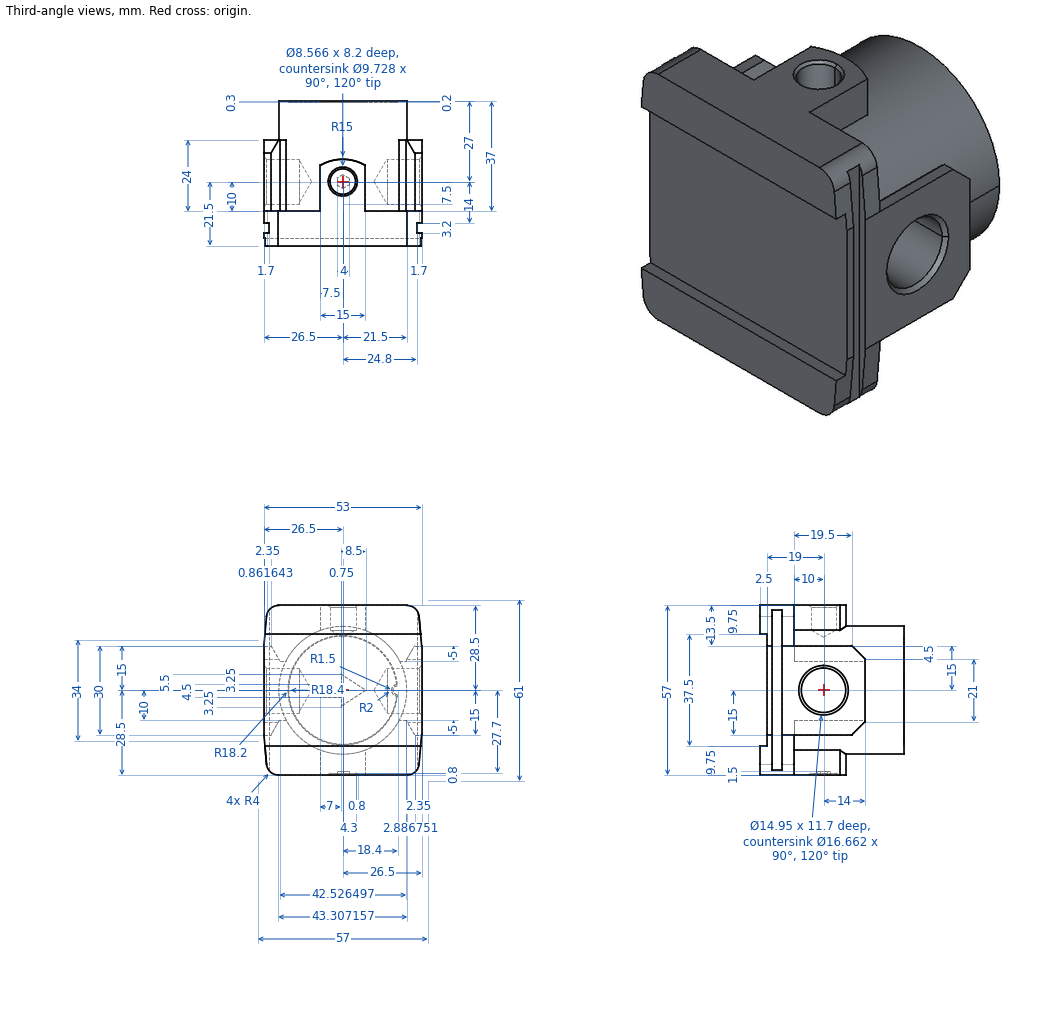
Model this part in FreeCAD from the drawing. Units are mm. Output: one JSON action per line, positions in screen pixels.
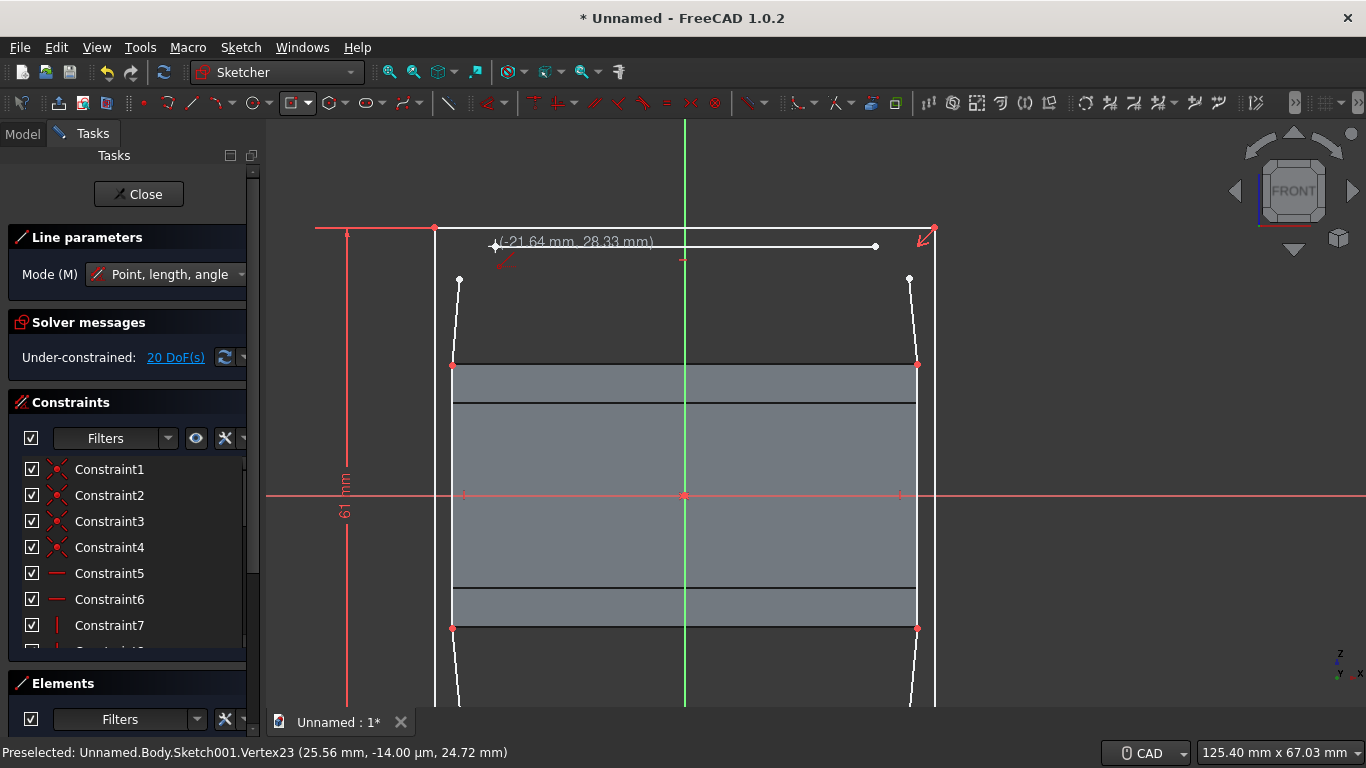
{"action": "left_click", "coordinate": [216, 104]}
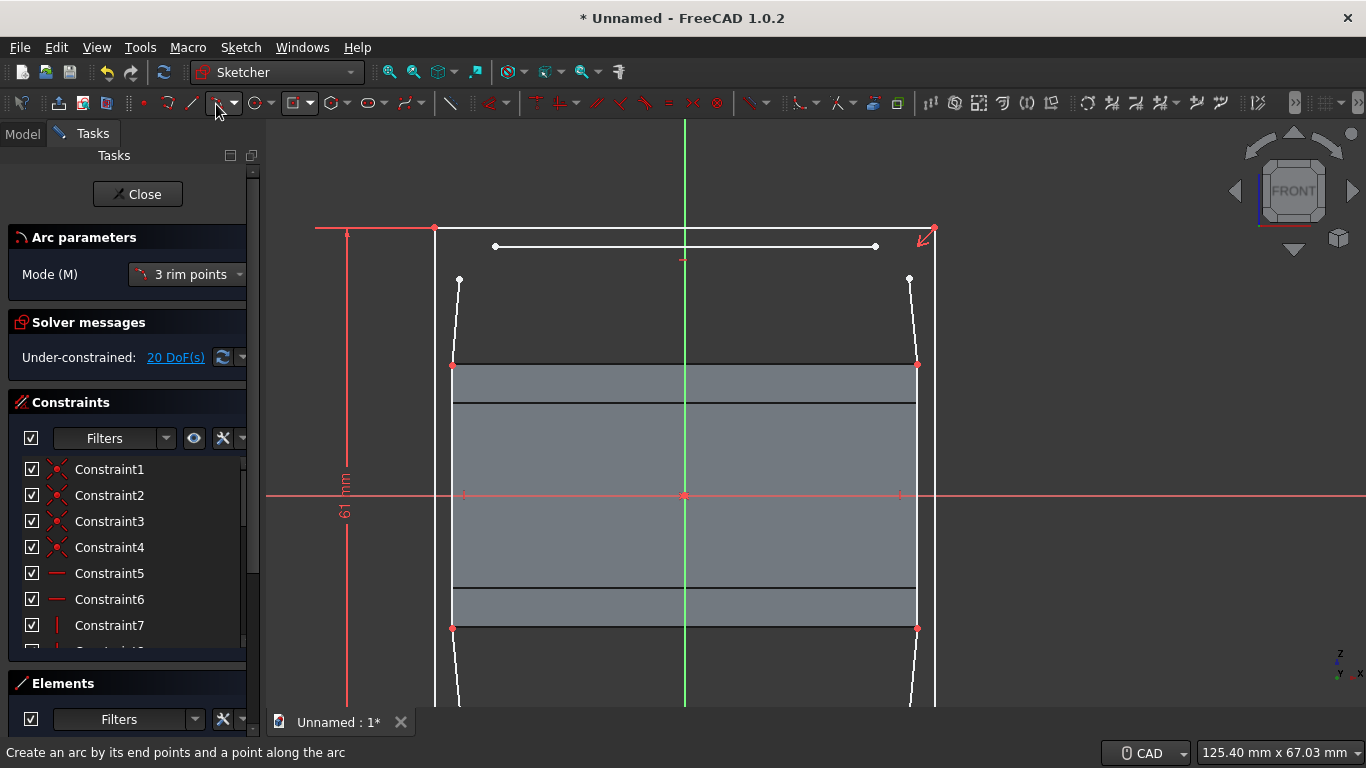
{"action": "scroll", "coordinate": [875, 245], "scroll_direction": "down", "scroll_amount": 2}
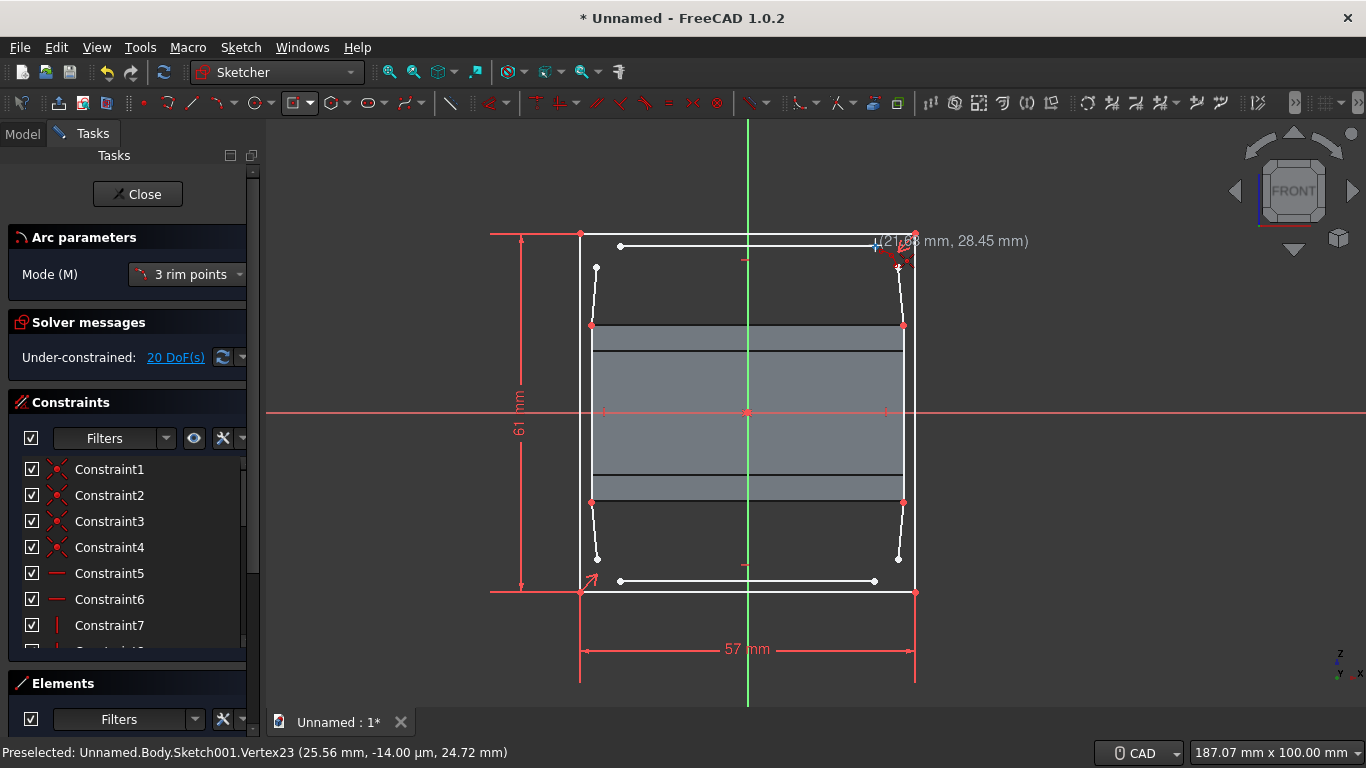
{"action": "left_click", "coordinate": [597, 560]}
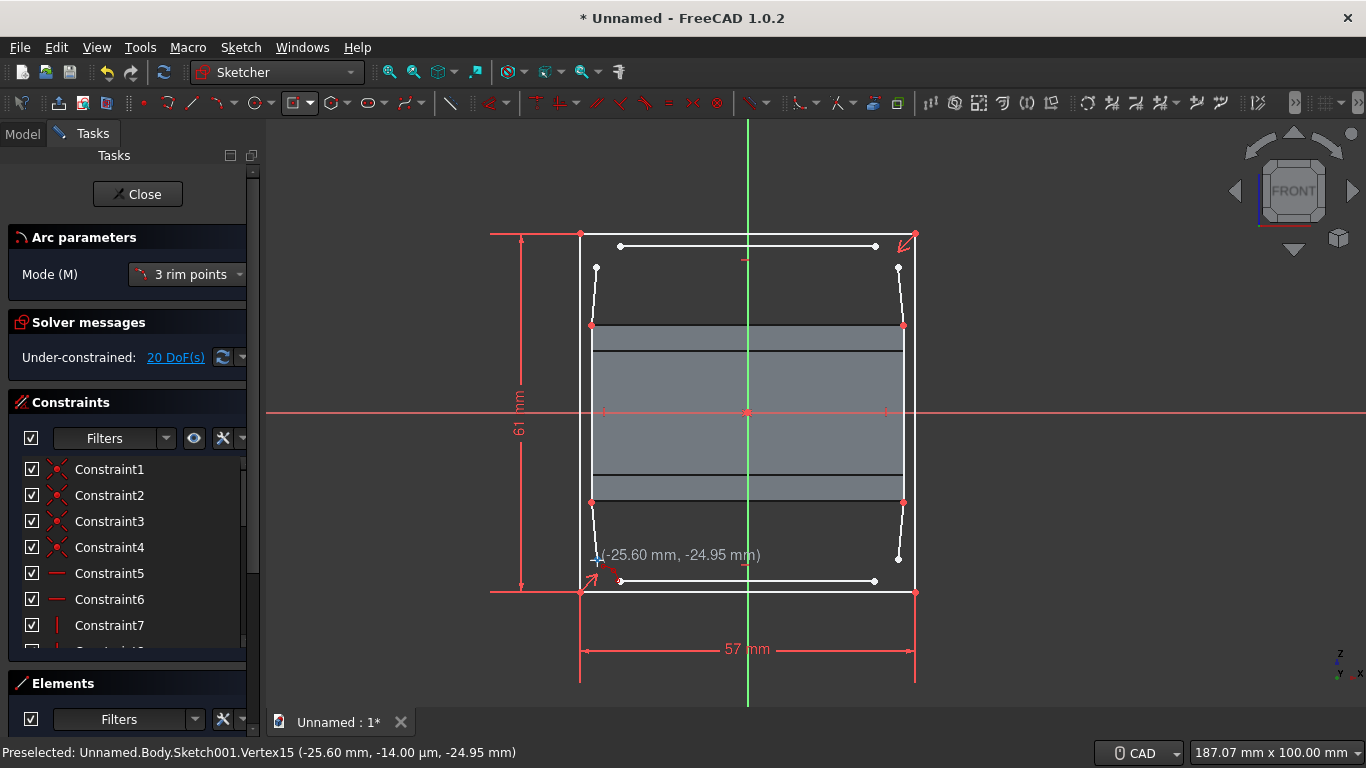
{"action": "scroll", "coordinate": [620, 581], "scroll_direction": "up", "scroll_amount": 2}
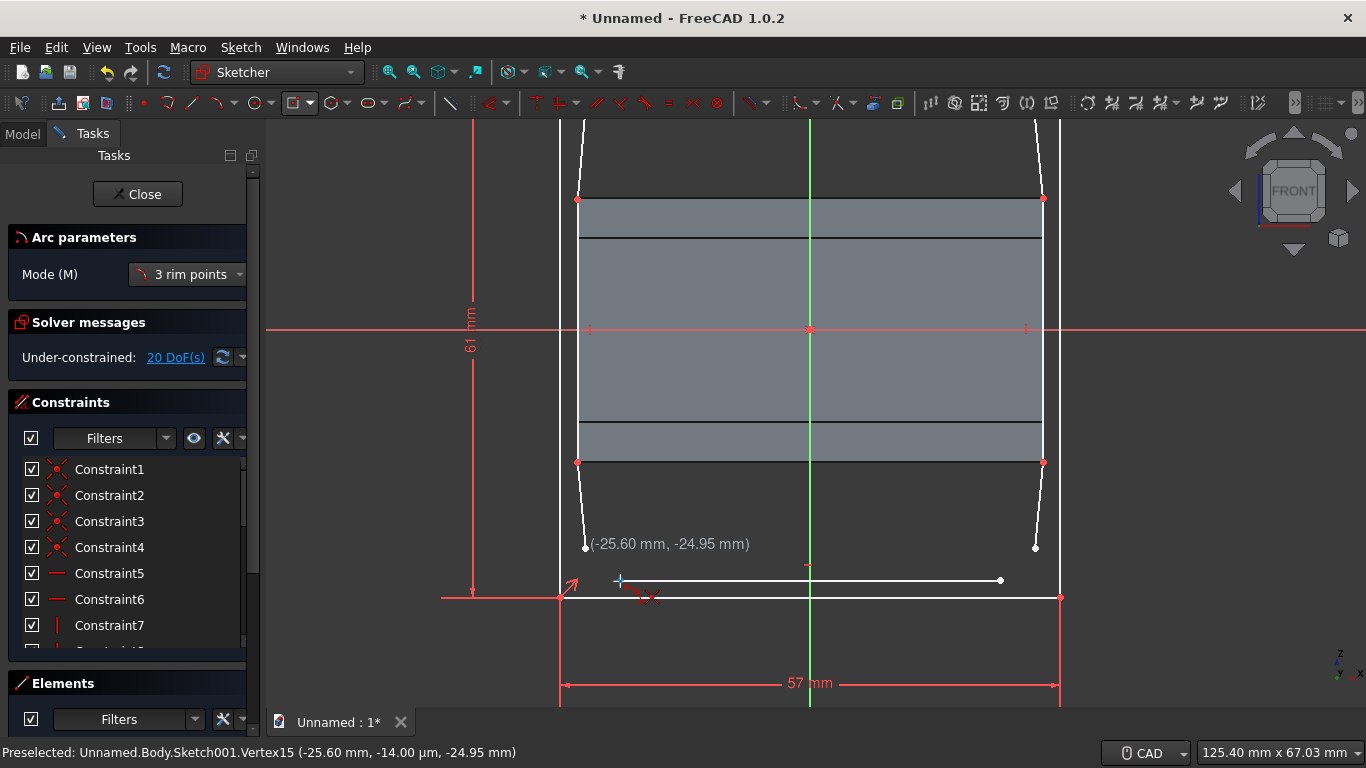
{"action": "left_click", "coordinate": [620, 581]}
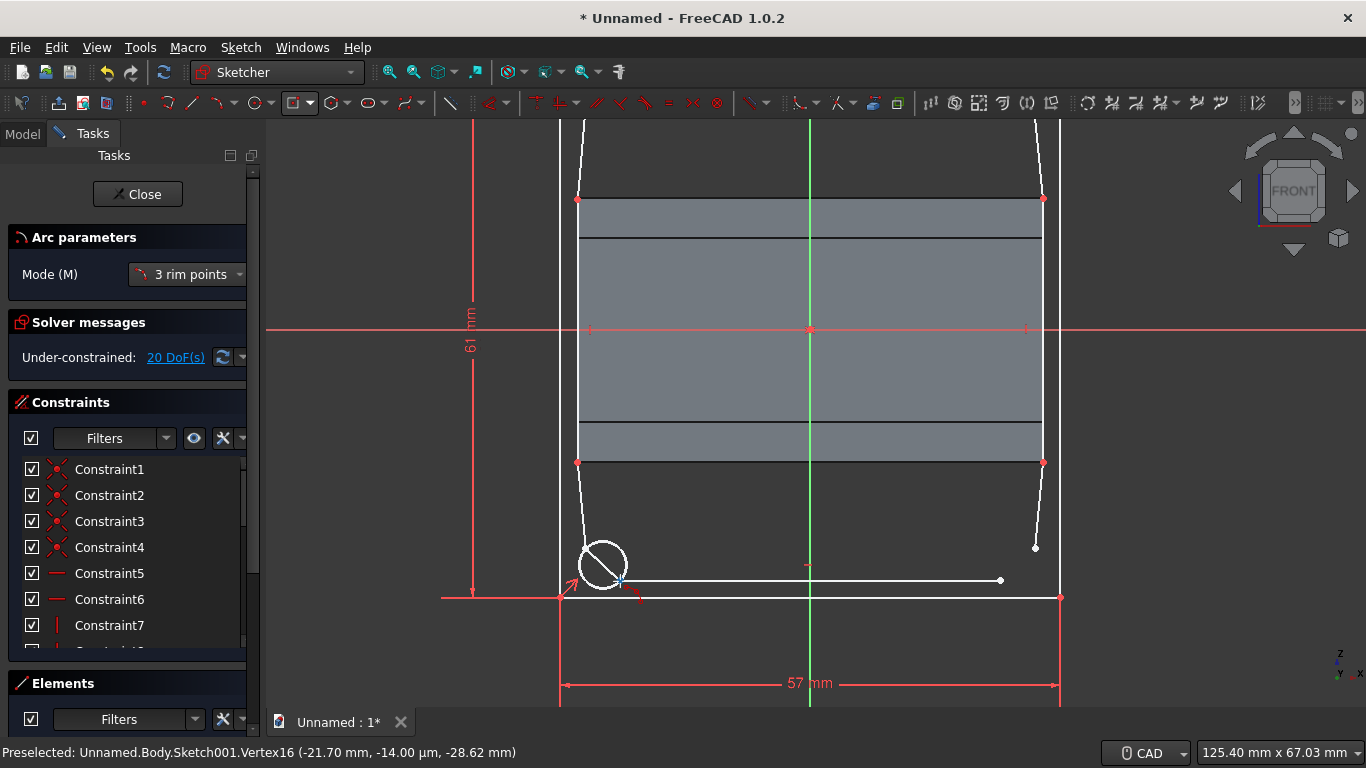
{"action": "scroll", "coordinate": [597, 571], "scroll_direction": "up", "scroll_amount": 3}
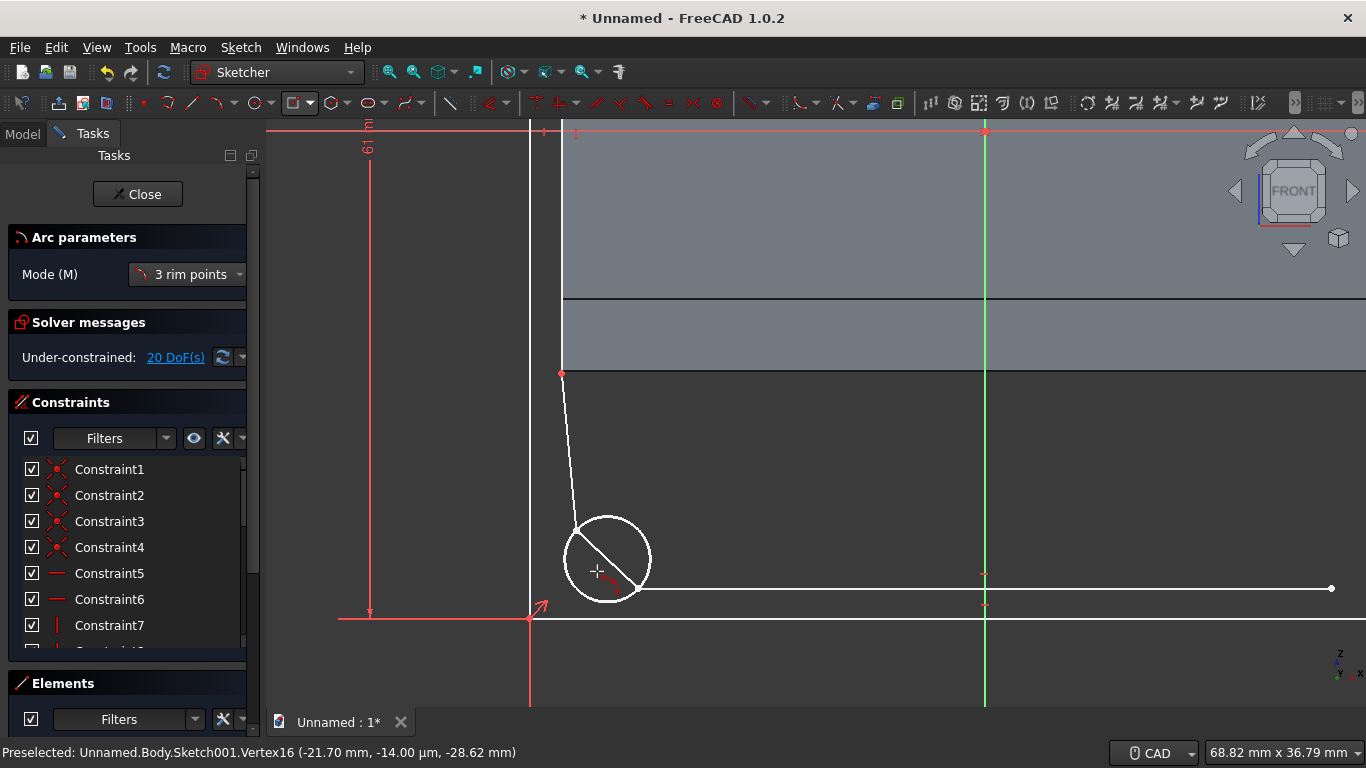
{"action": "left_click", "coordinate": [596, 570]}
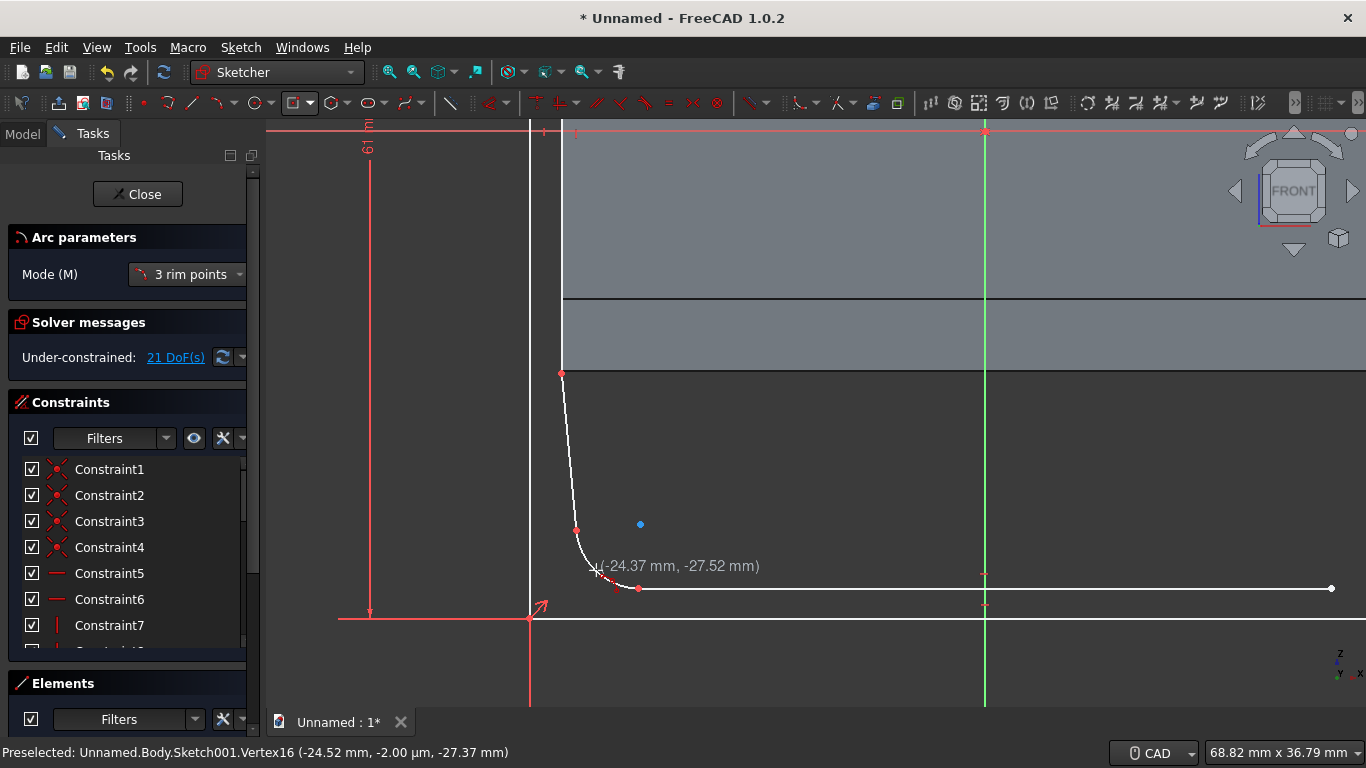
{"action": "scroll", "coordinate": [609, 577], "scroll_direction": "down", "scroll_amount": 5}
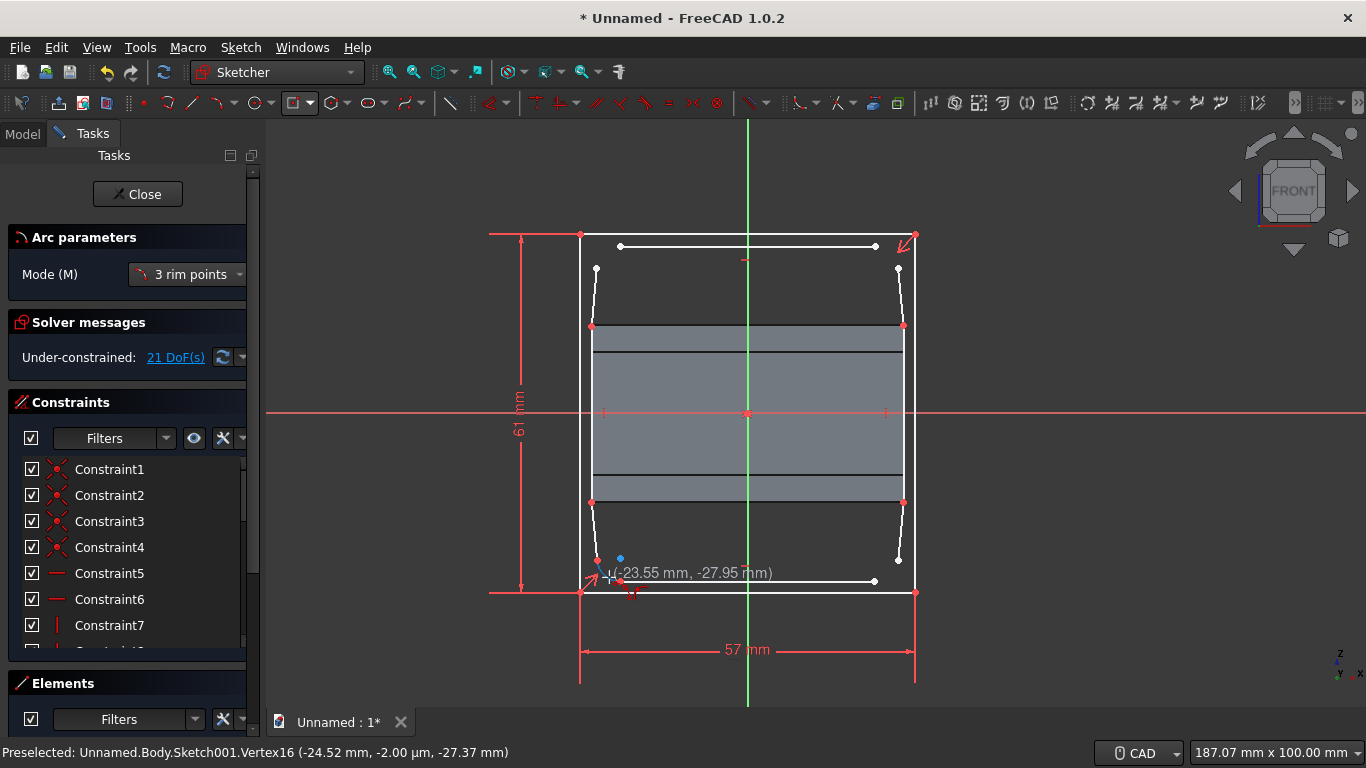
{"action": "scroll", "coordinate": [875, 581], "scroll_direction": "up", "scroll_amount": 2}